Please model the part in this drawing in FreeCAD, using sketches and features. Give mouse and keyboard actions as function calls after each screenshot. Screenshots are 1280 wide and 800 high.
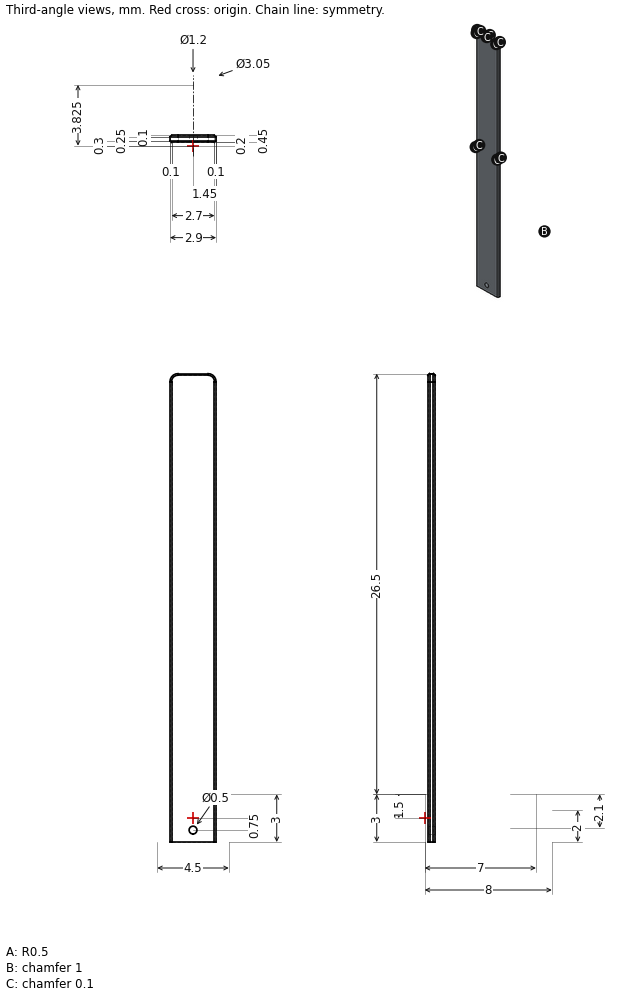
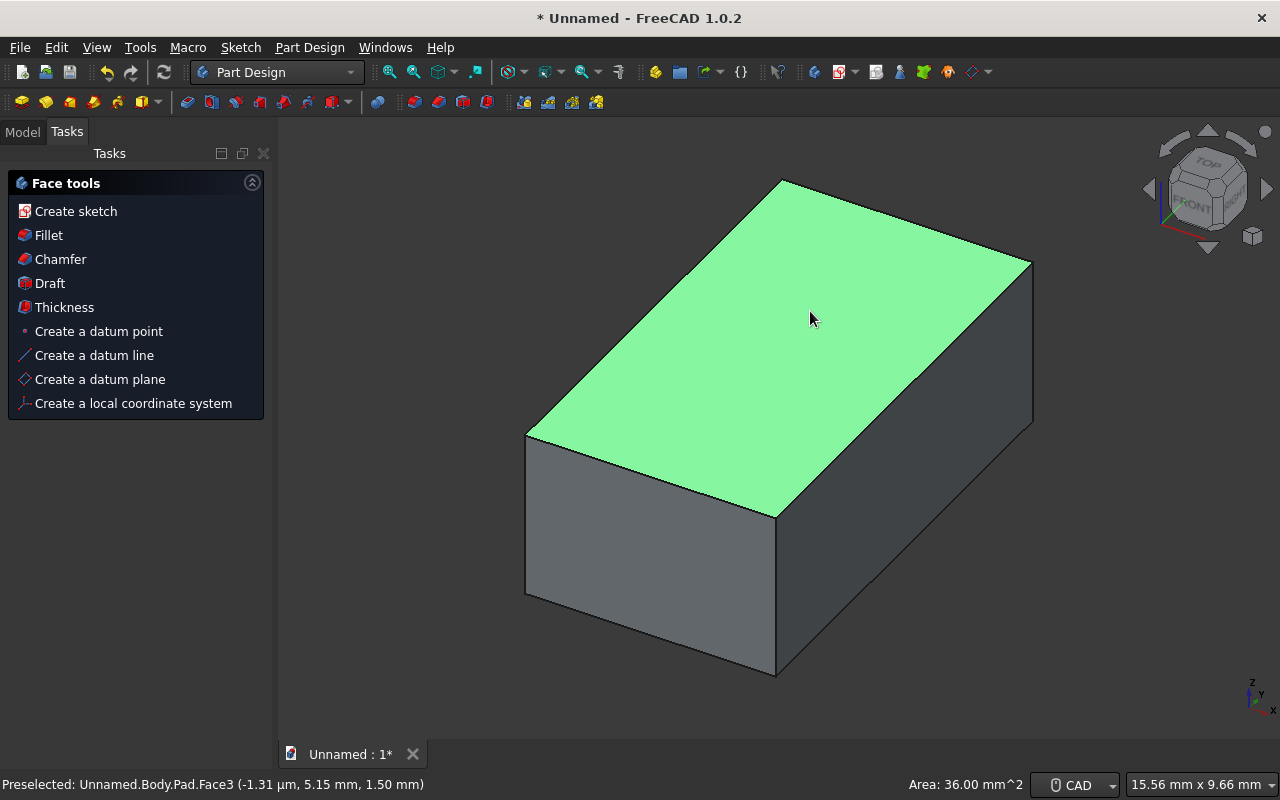
click(840, 72)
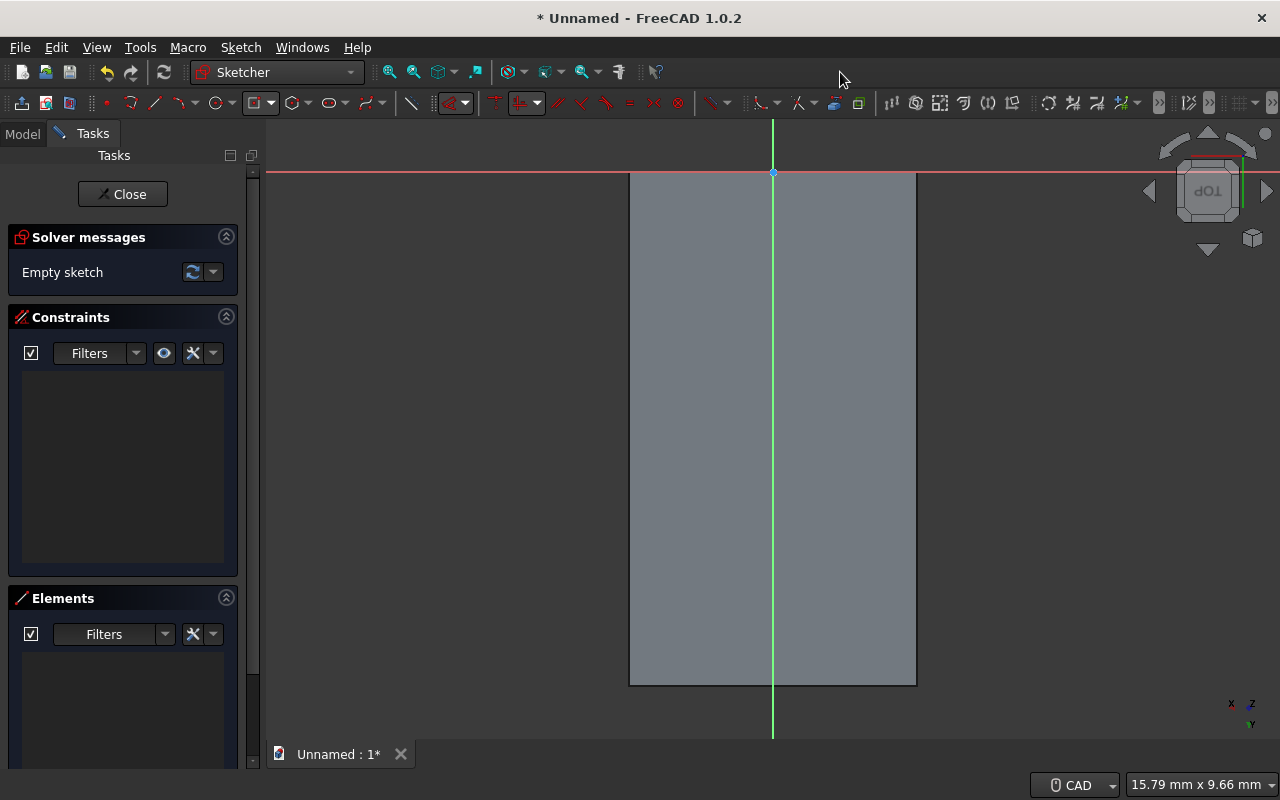
scroll(803, 147, up, 6)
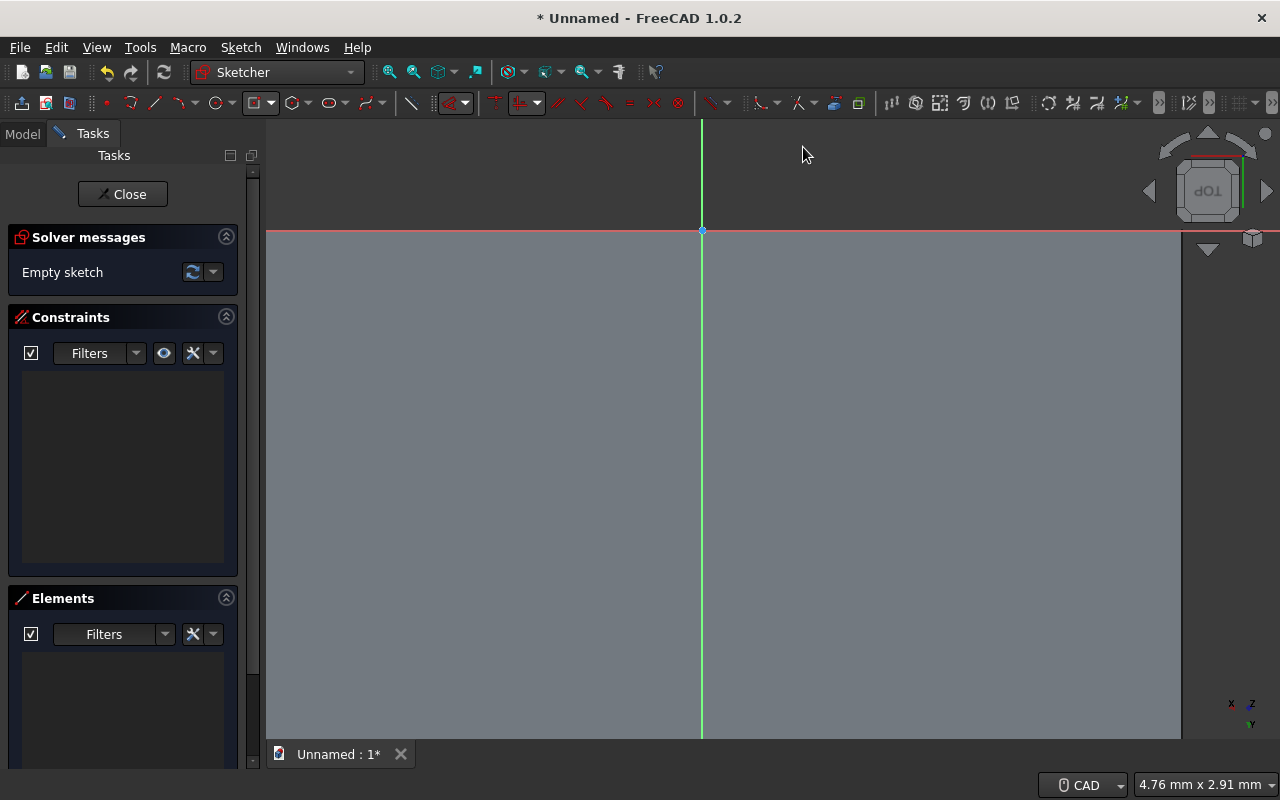
key(g)
key(r)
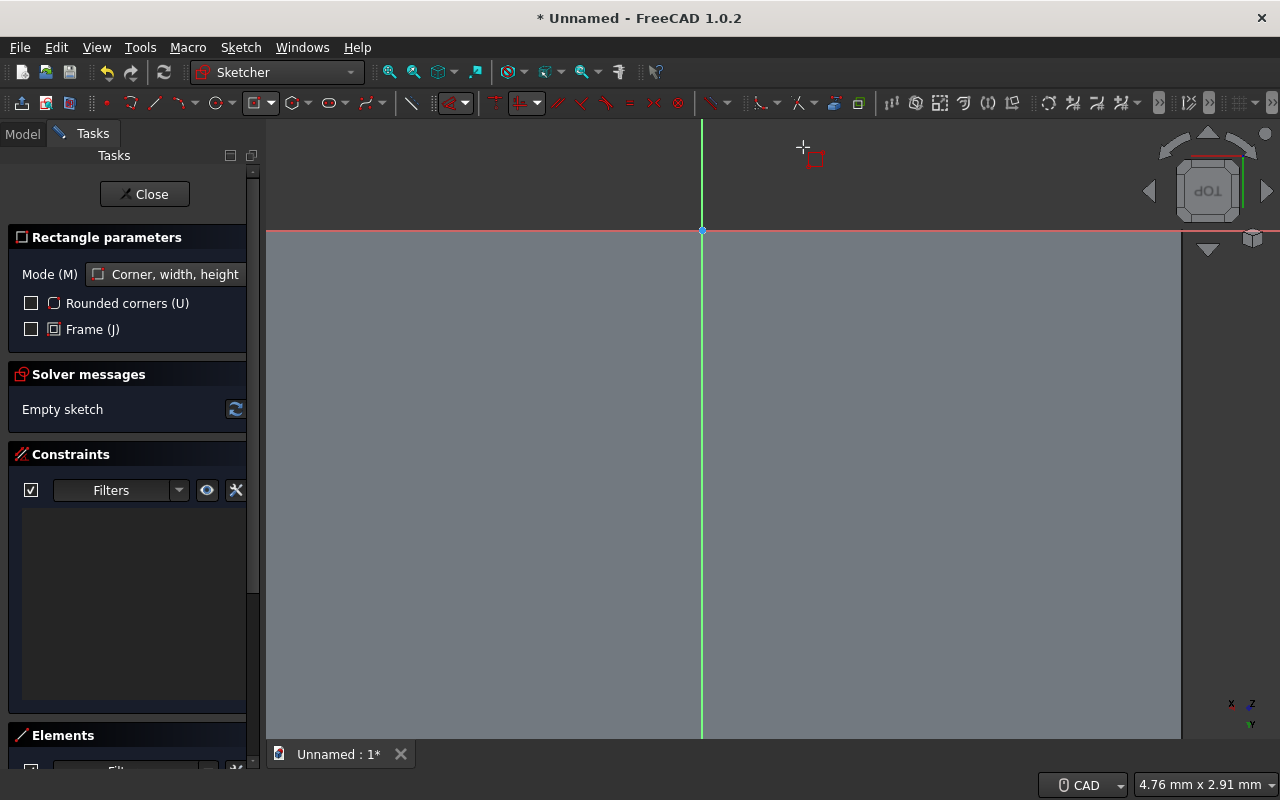
click(393, 273)
click(1011, 369)
key(Escape)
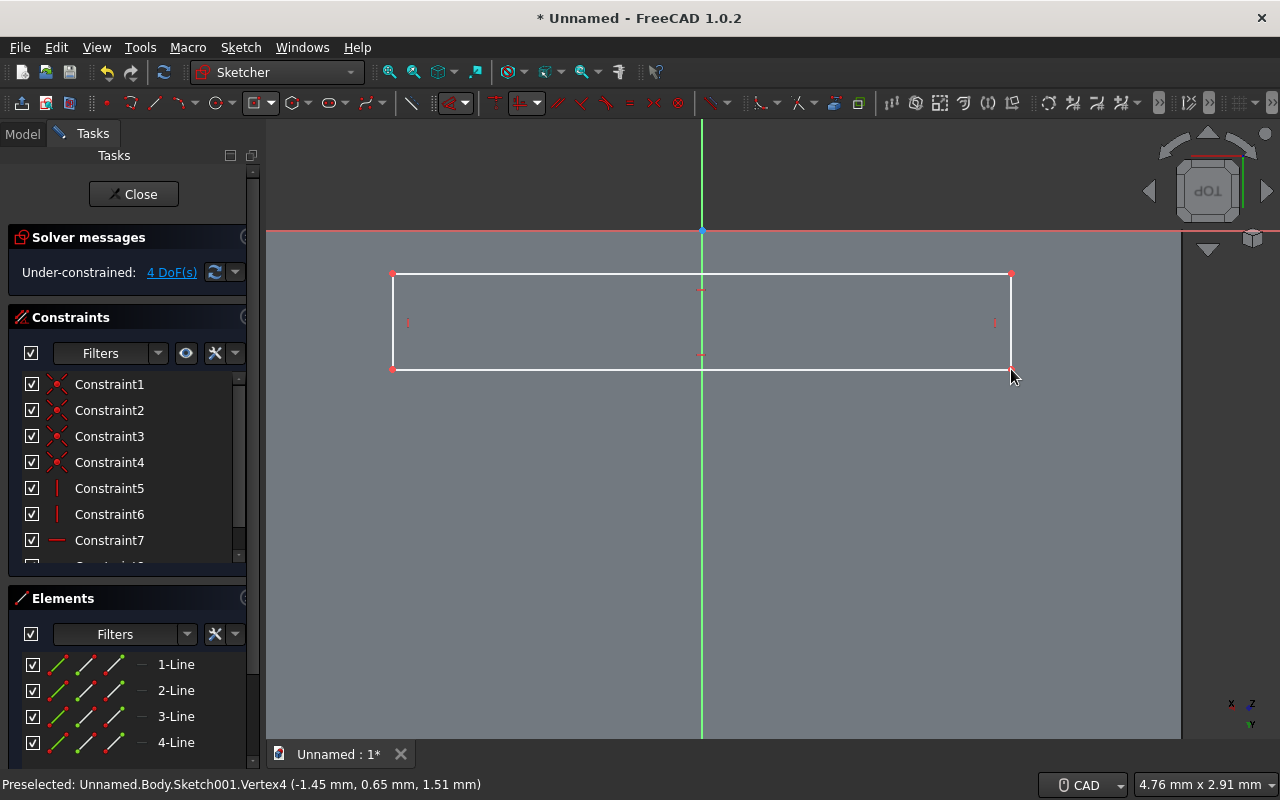
key(d)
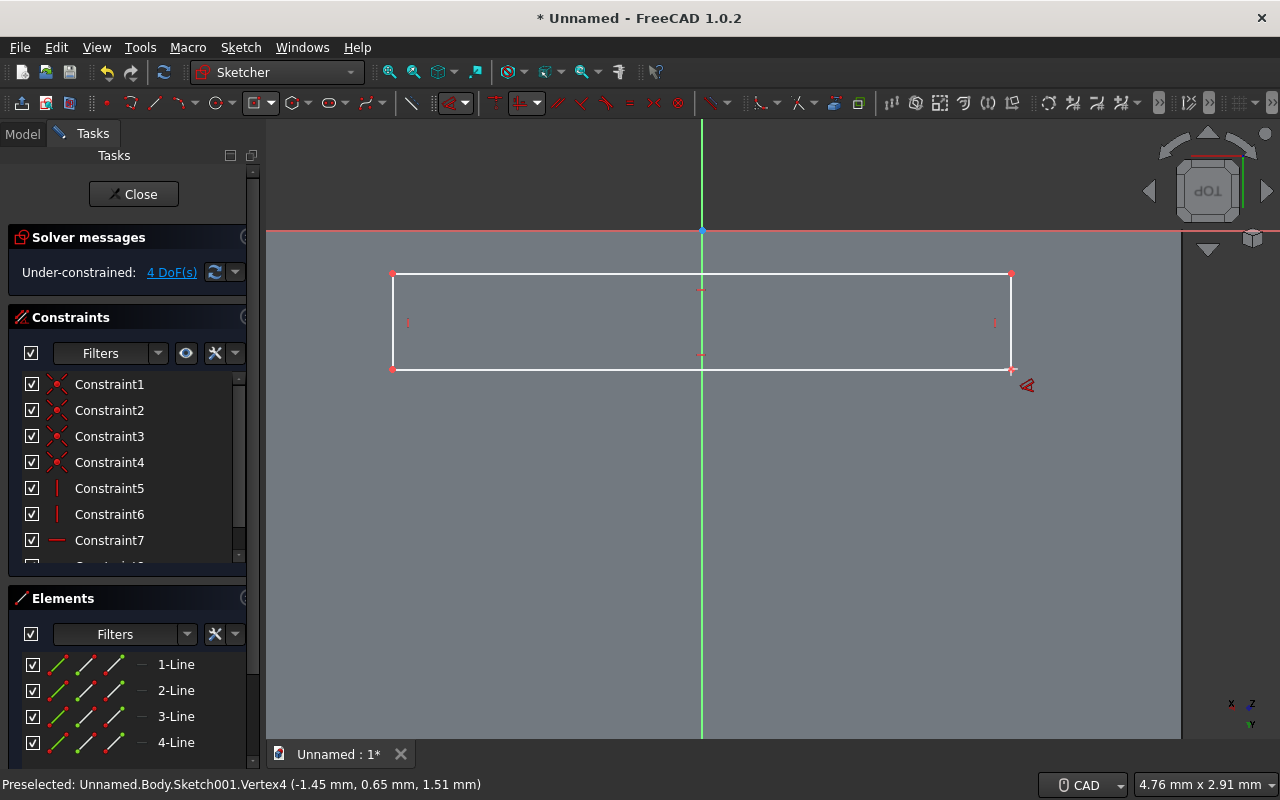
click(578, 370)
click(560, 404)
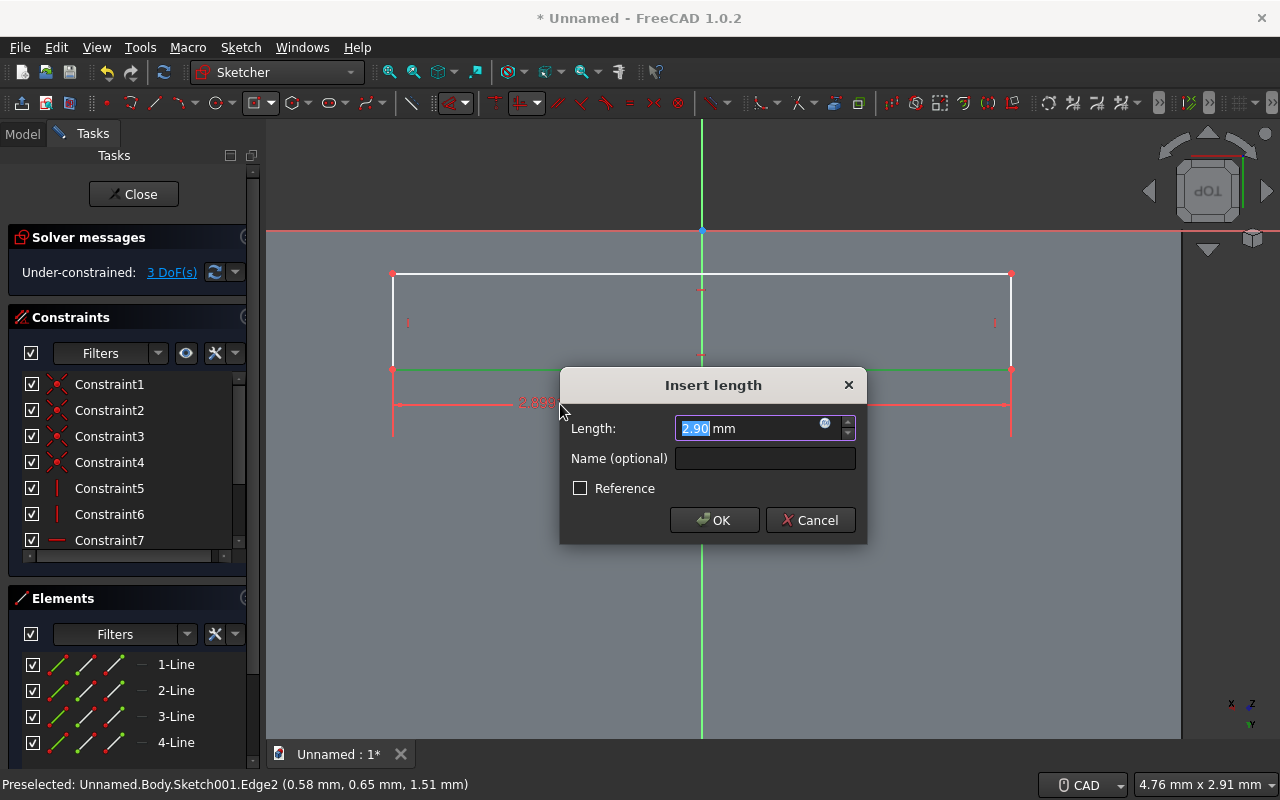
text(2.9)
key(Return)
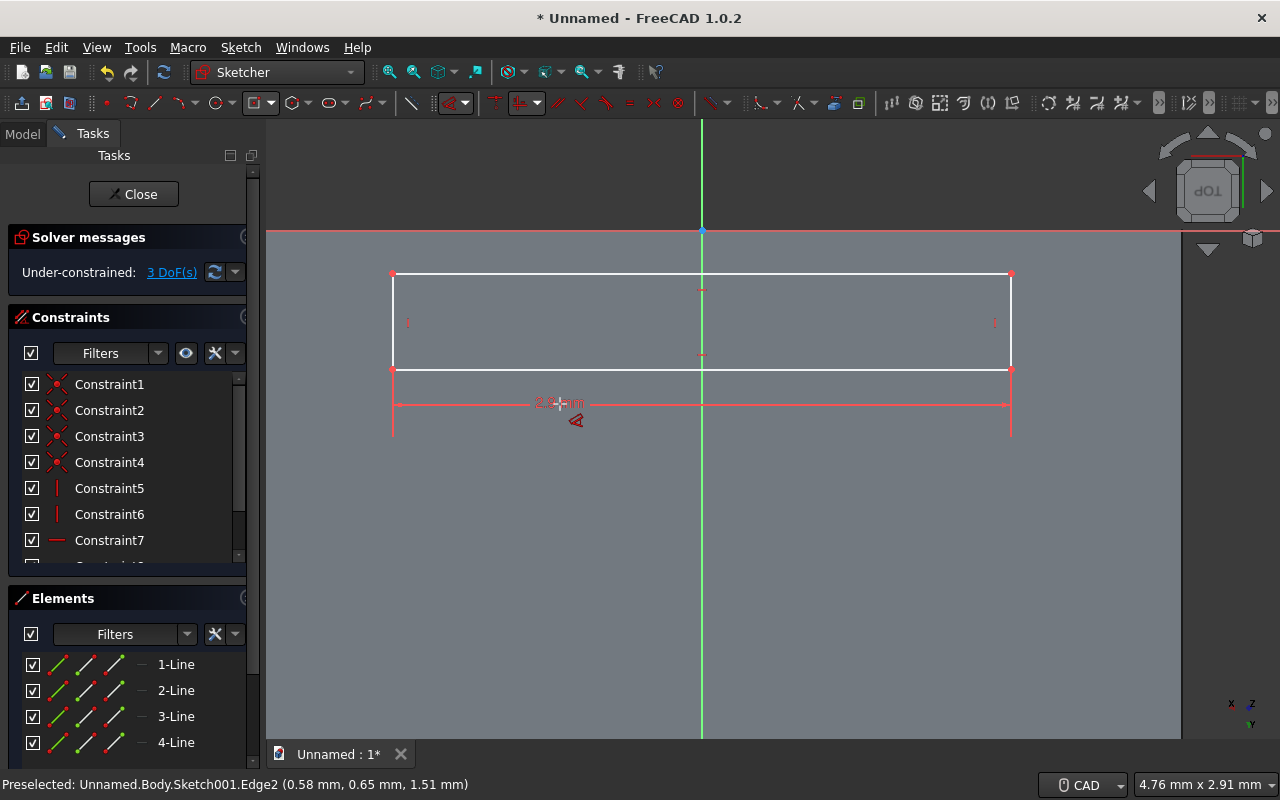
click(393, 303)
click(359, 322)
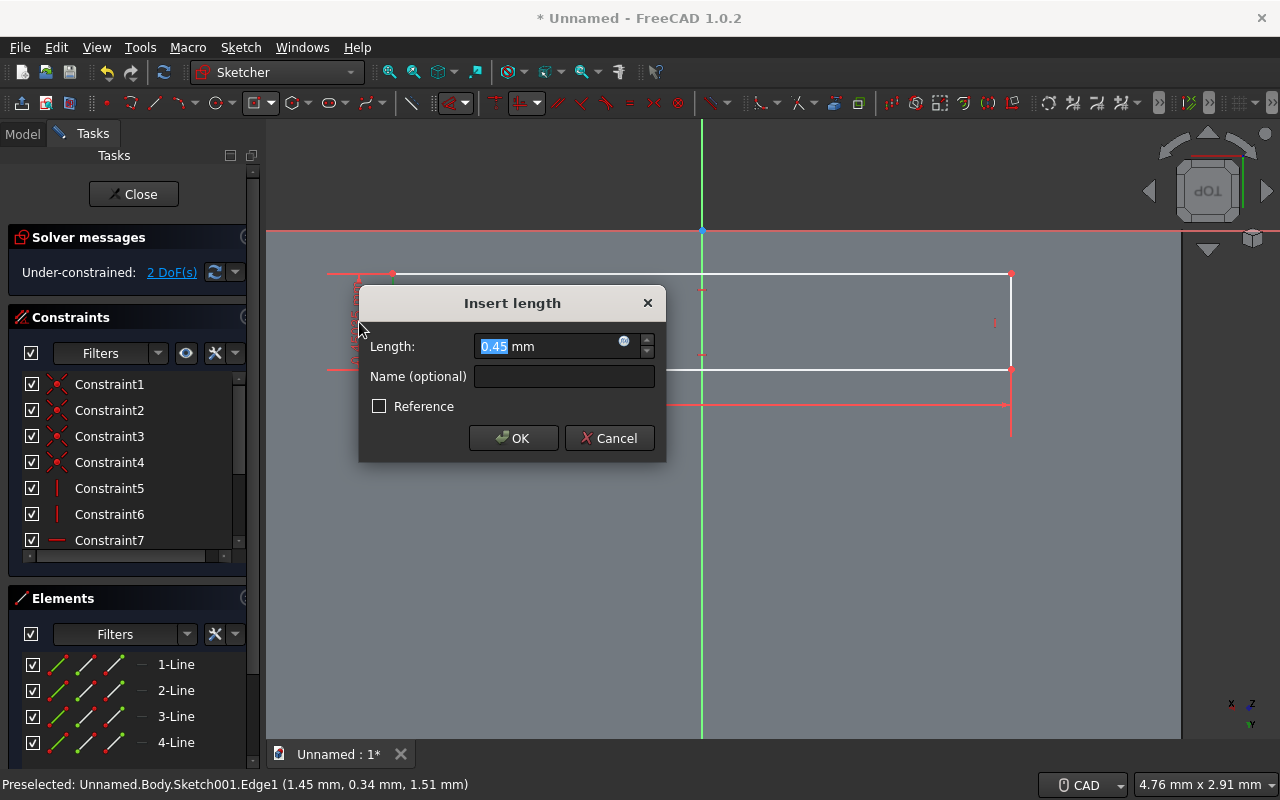
text(0.45)
key(Return)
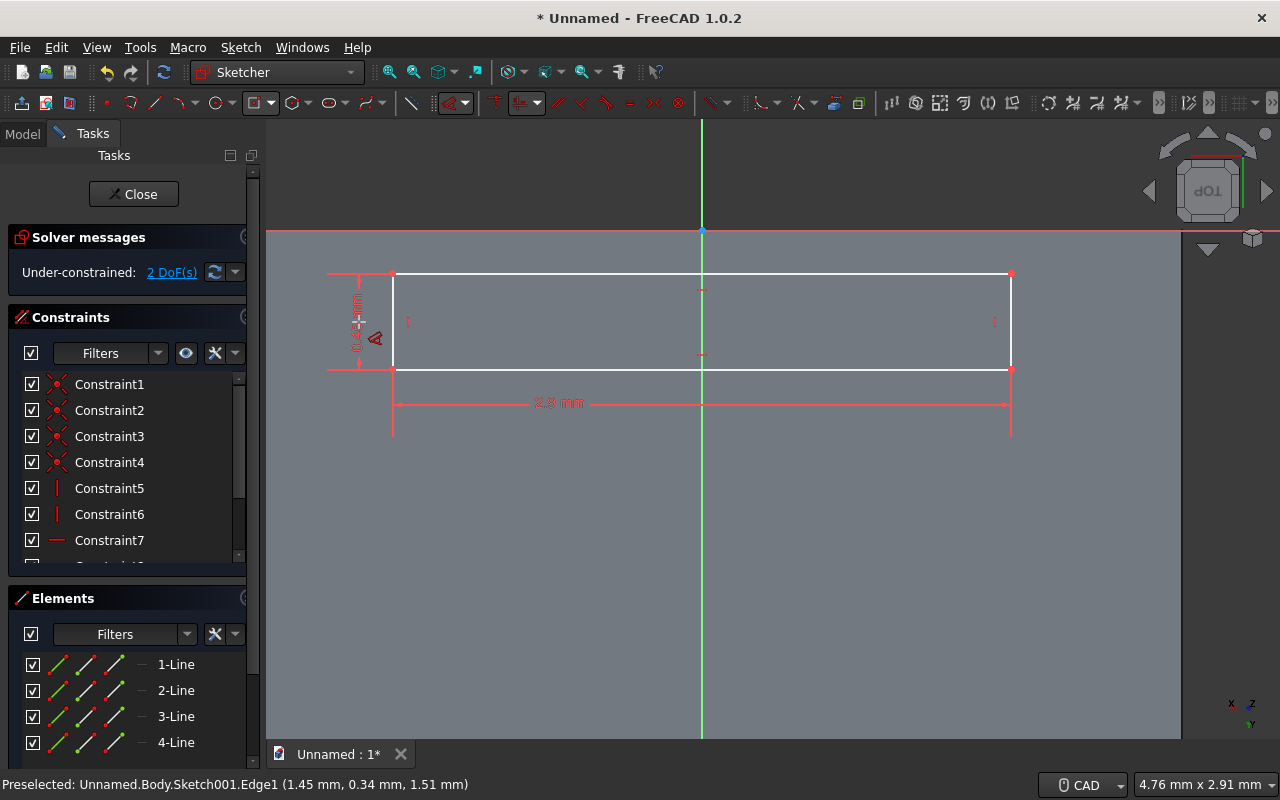
click(393, 274)
click(359, 252)